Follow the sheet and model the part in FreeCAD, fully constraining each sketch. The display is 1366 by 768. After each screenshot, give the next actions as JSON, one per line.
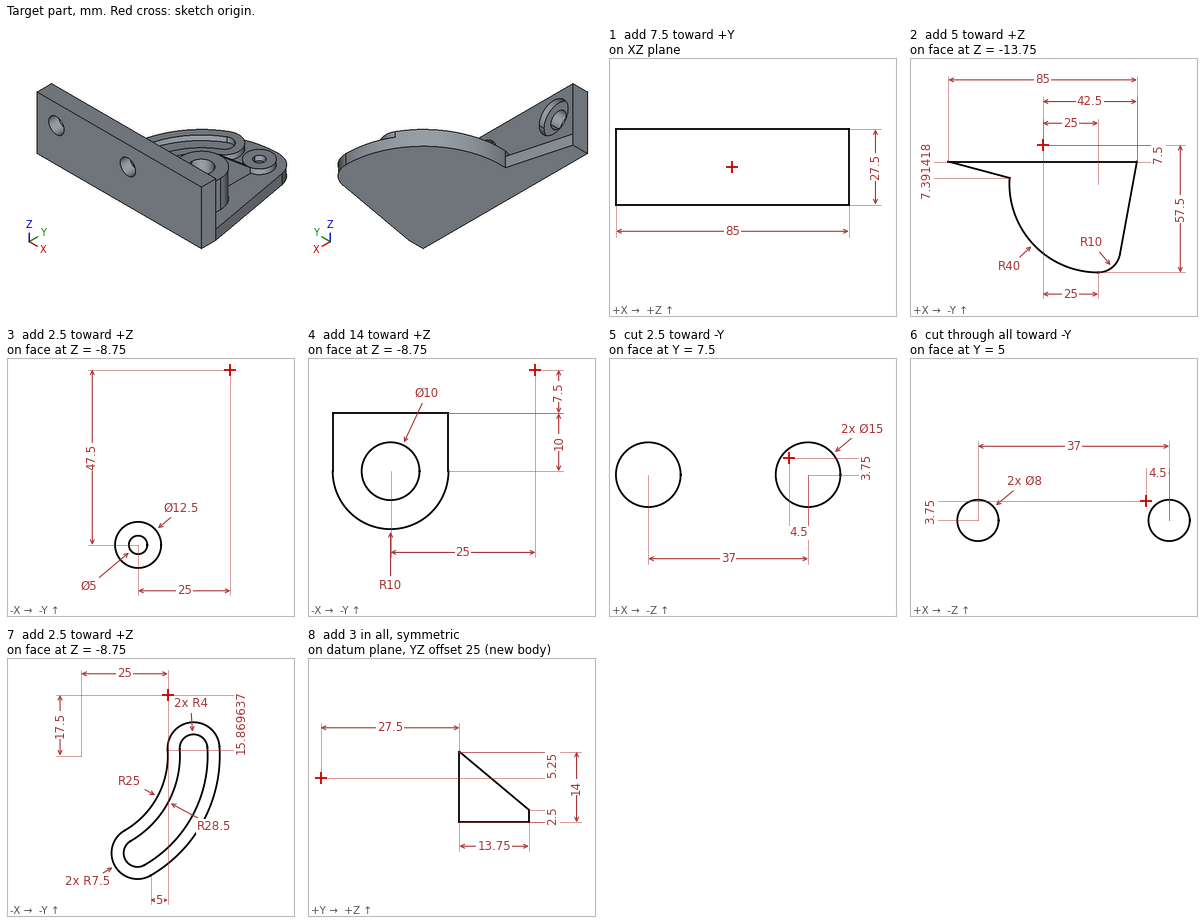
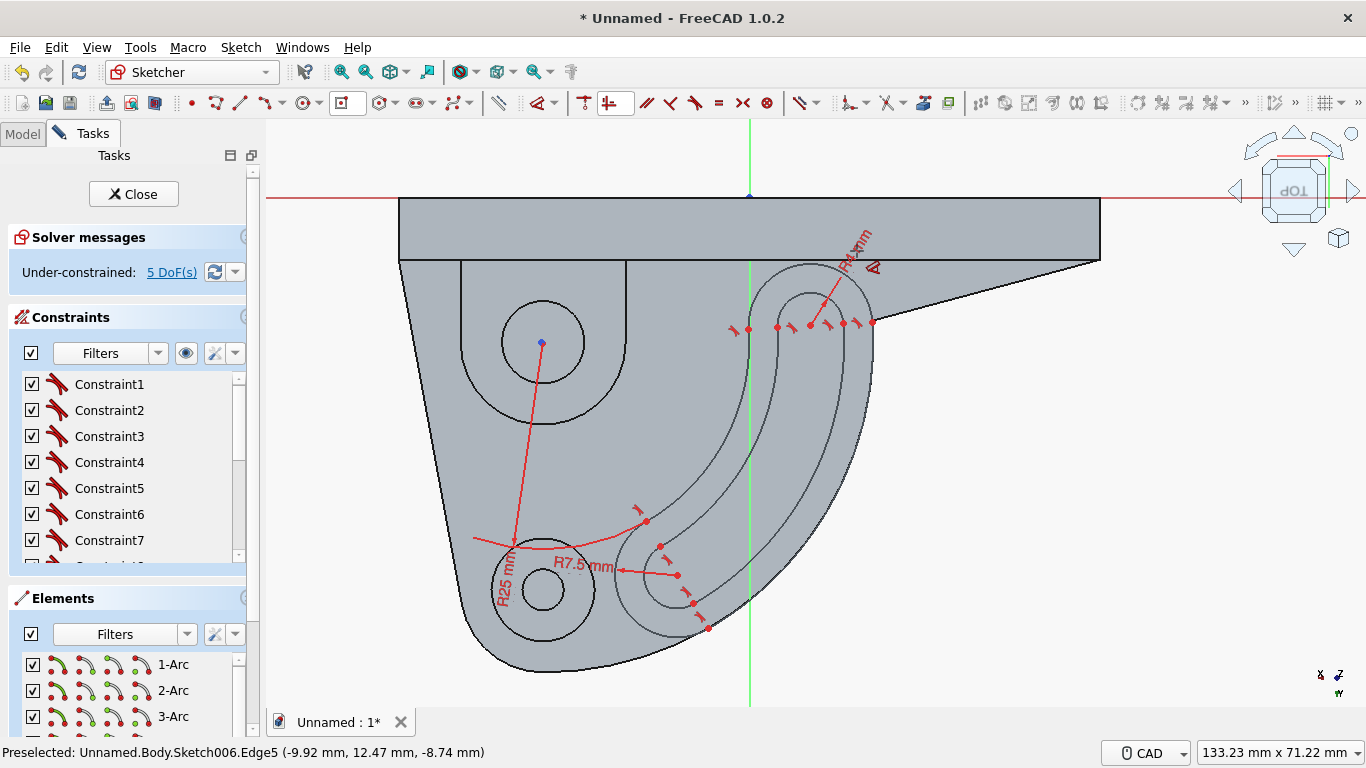
{"action": "left_click", "coordinate": [720, 497]}
{"action": "left_click", "coordinate": [804, 399]}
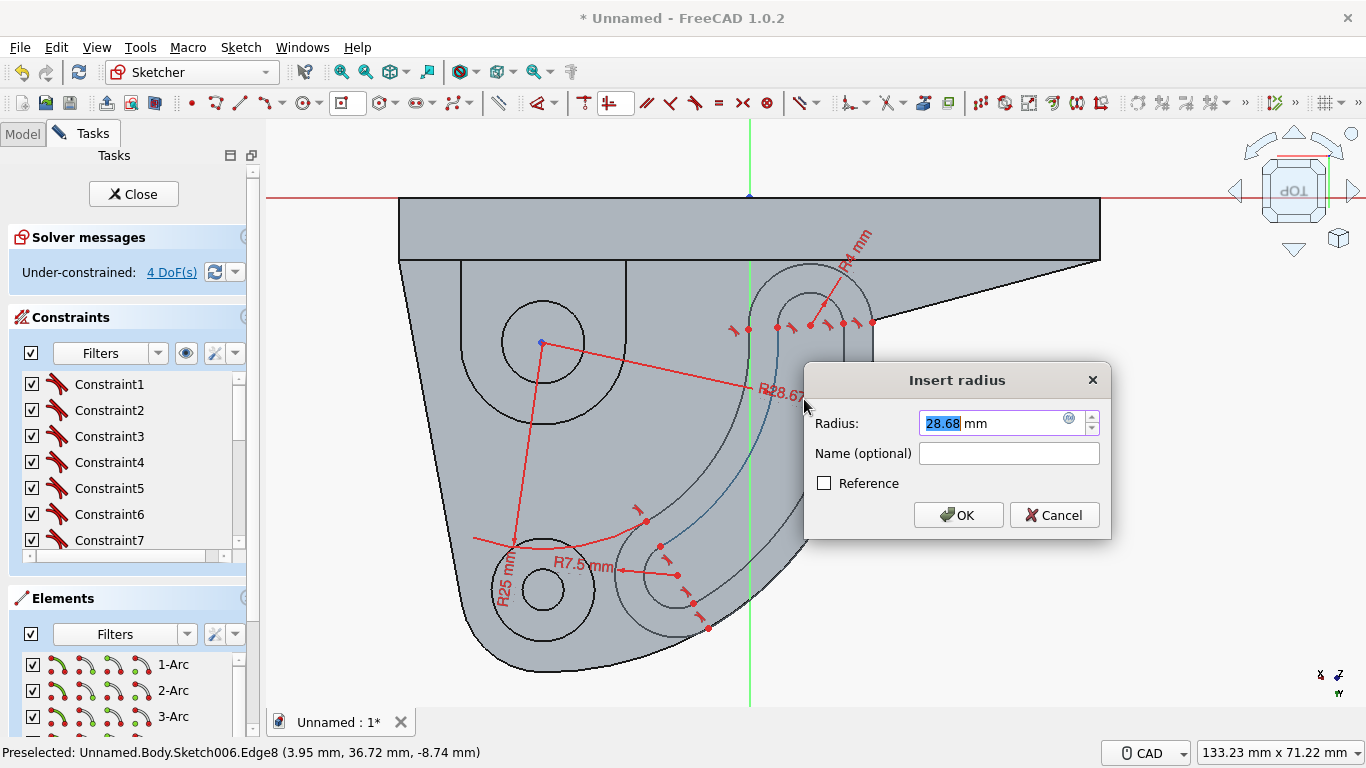
{"action": "type", "text": "28.5"}
{"action": "key", "text": "Return"}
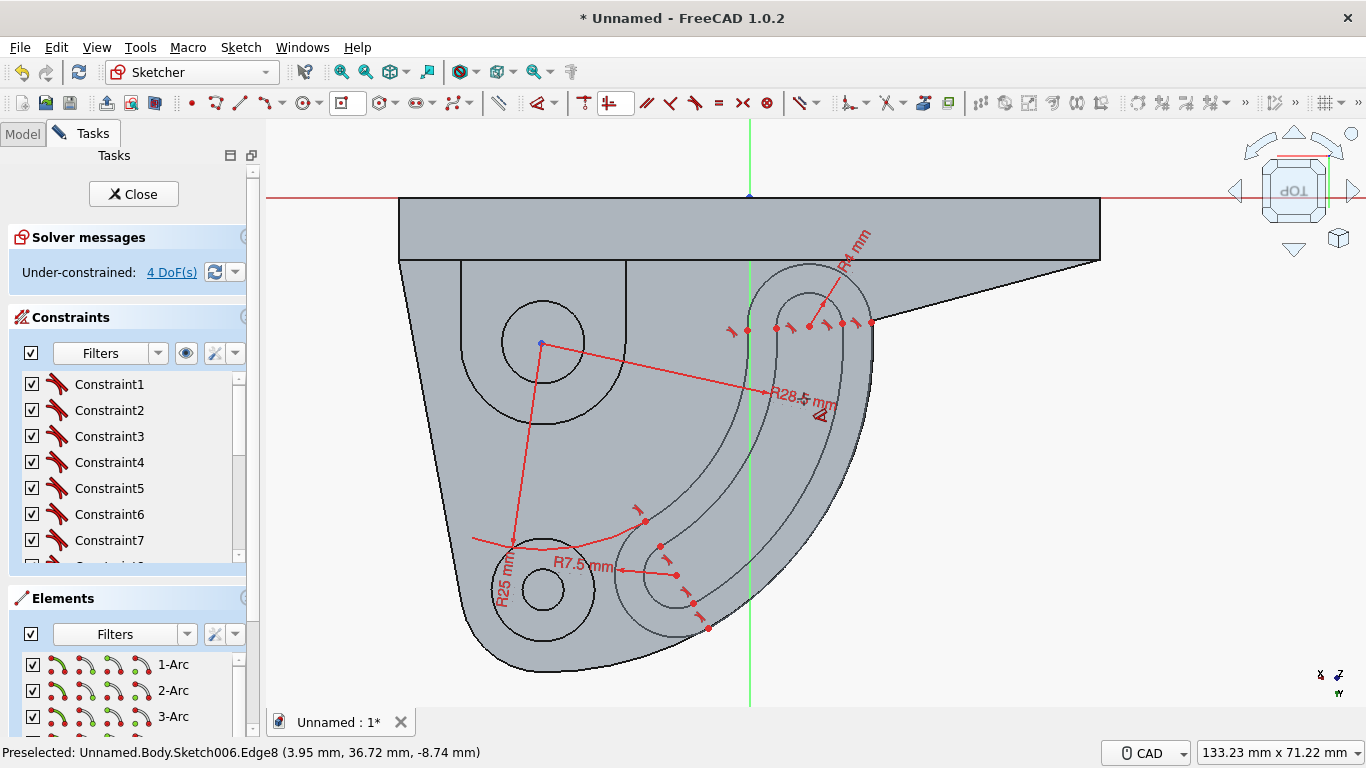
{"action": "left_click", "coordinate": [708, 629]}
{"action": "left_click", "coordinate": [729, 663]}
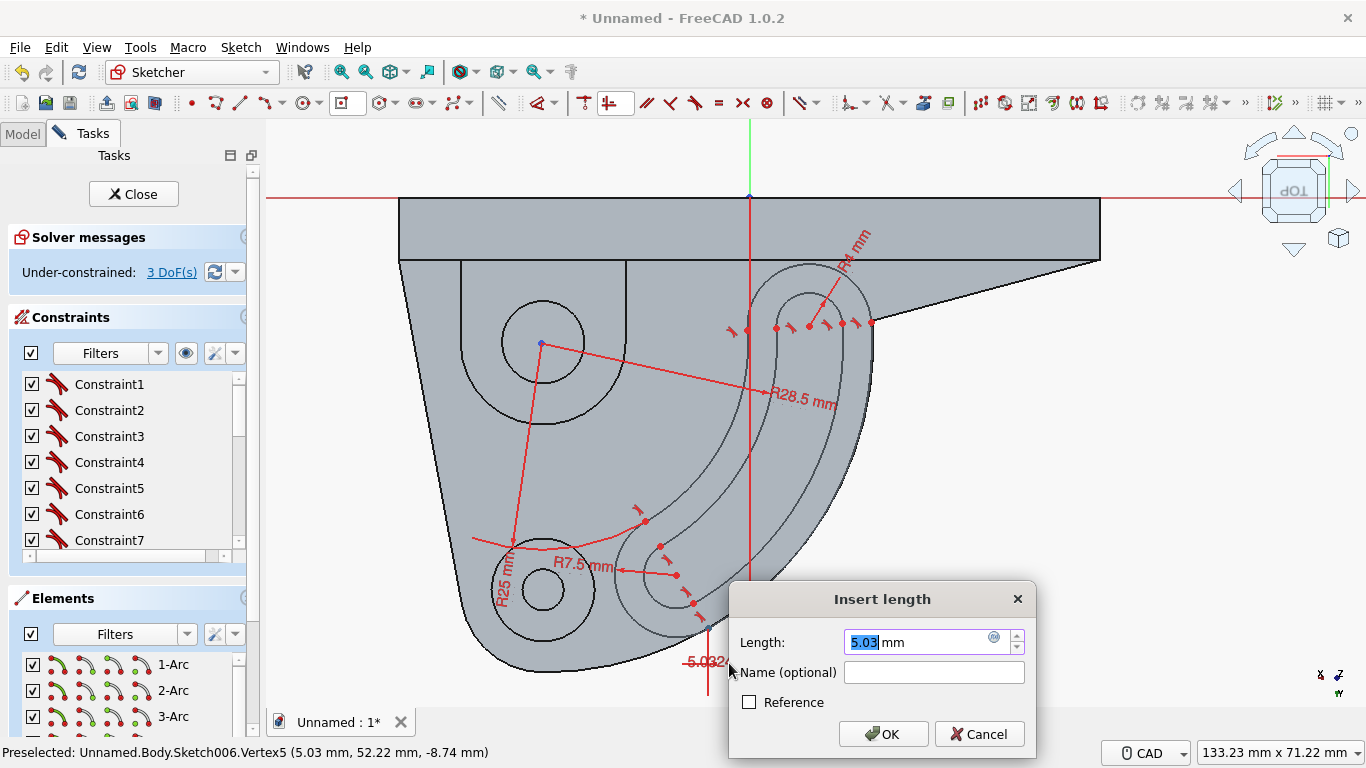
{"action": "type", "text": "5"}
{"action": "key", "text": "Return"}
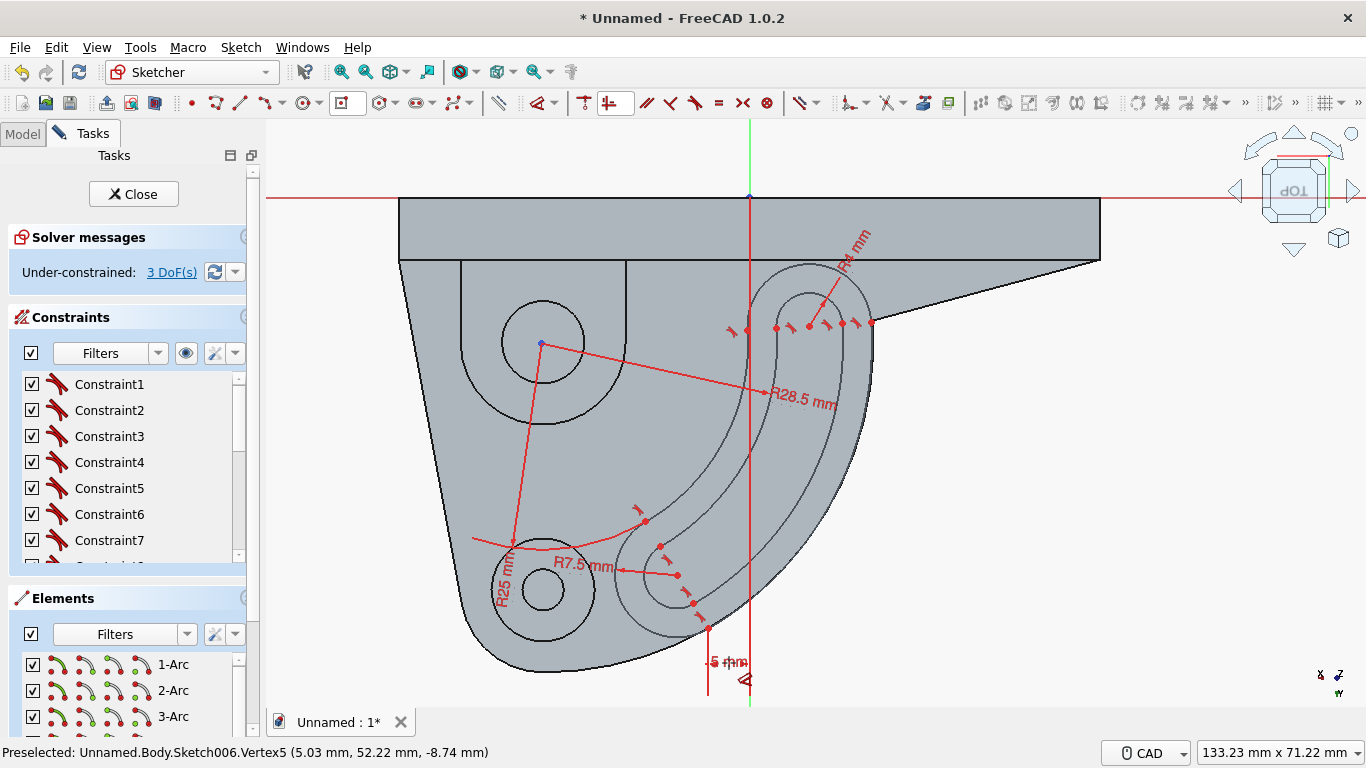
{"action": "left_click", "coordinate": [542, 344]}
{"action": "left_click", "coordinate": [646, 164]}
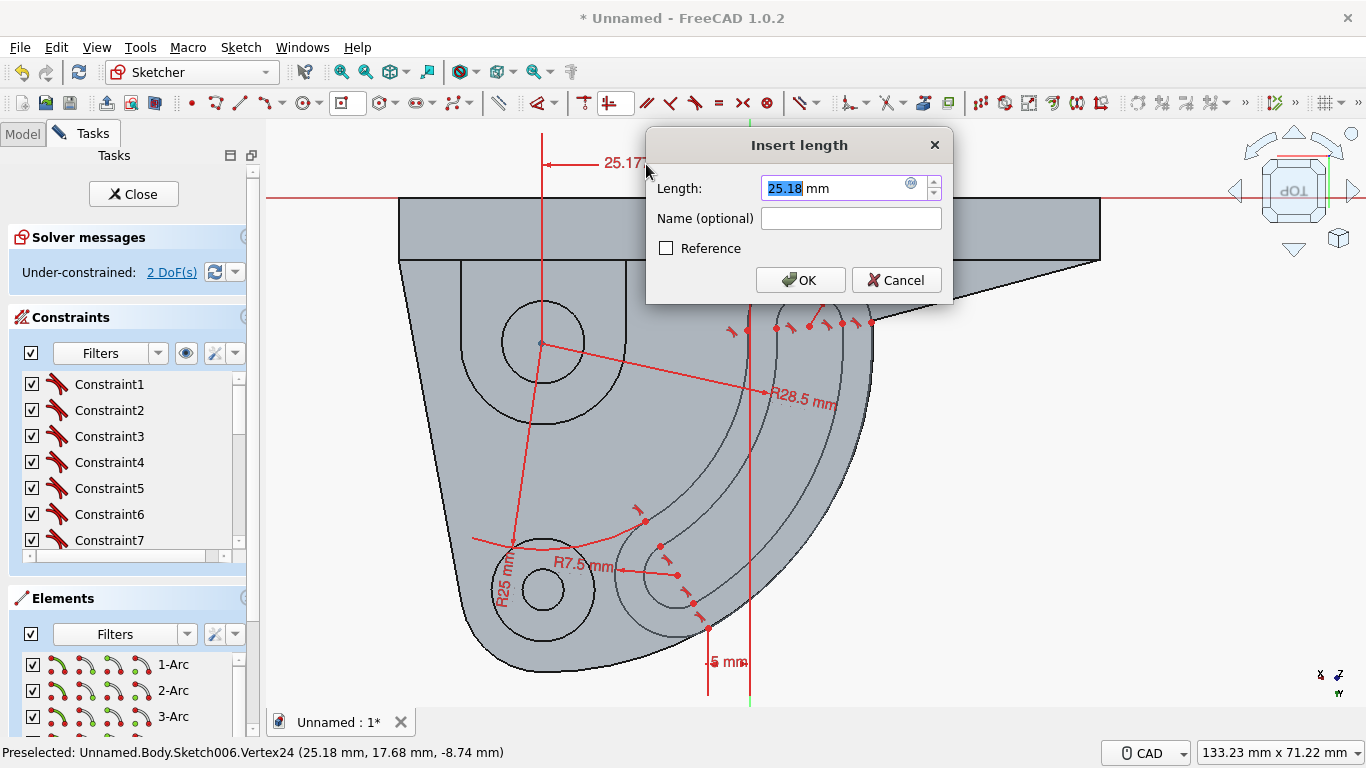
{"action": "type", "text": "25"}
{"action": "key", "text": "Return"}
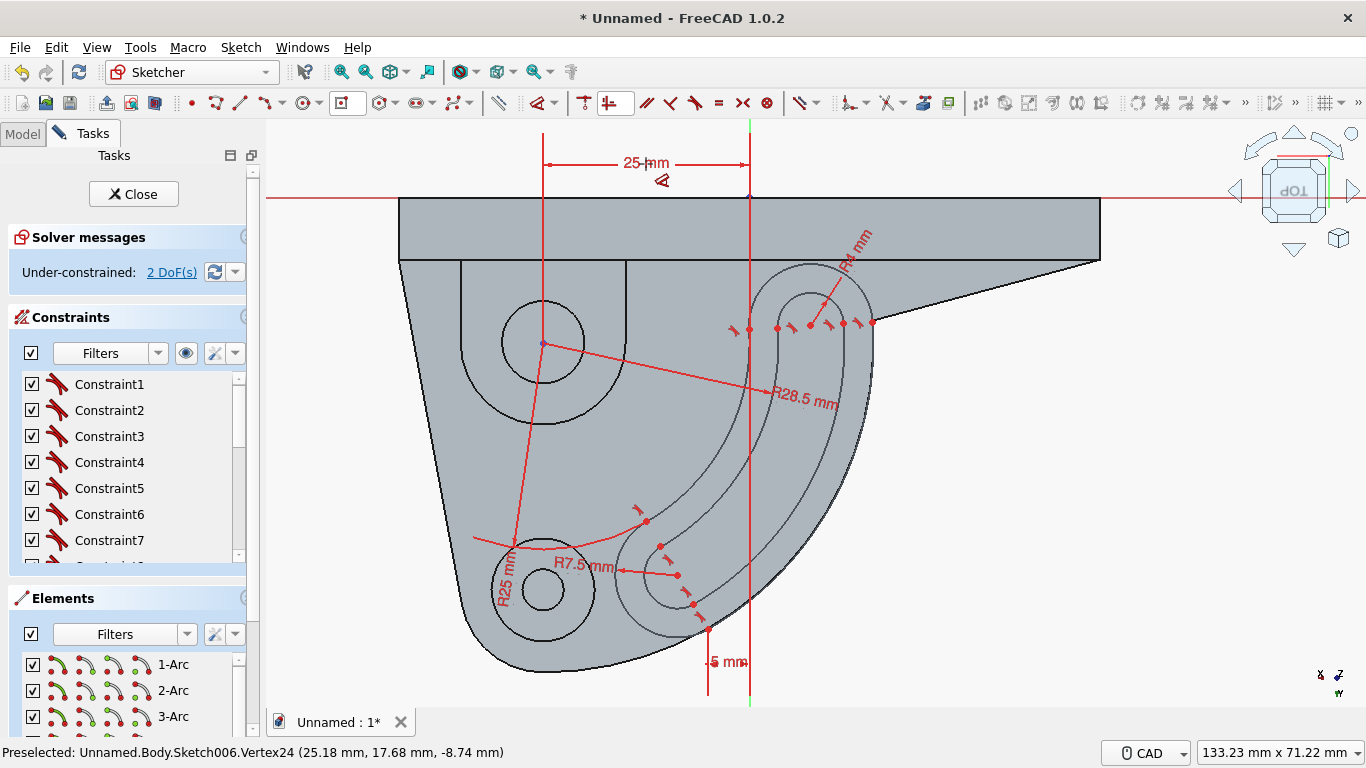
{"action": "left_click", "coordinate": [543, 343]}
{"action": "left_click", "coordinate": [509, 270]}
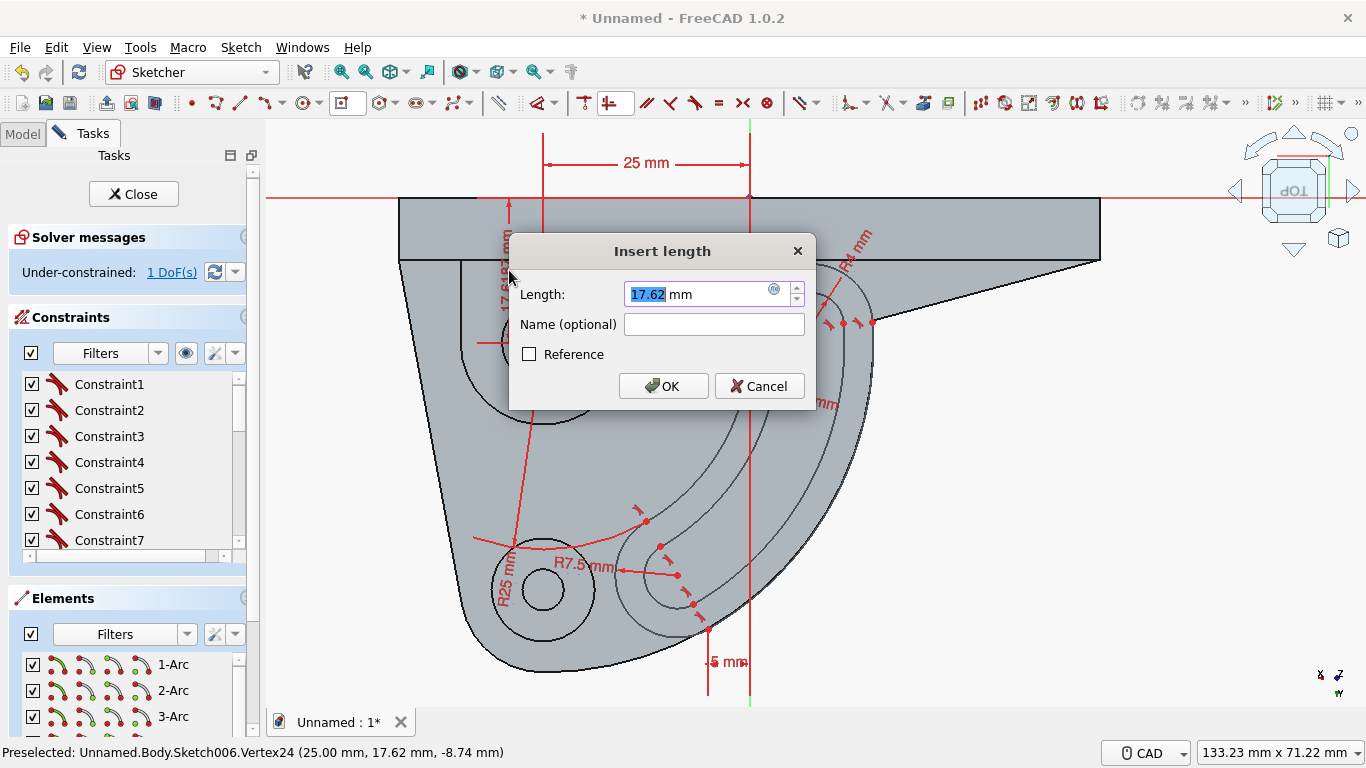
{"action": "type", "text": "17.5"}
{"action": "key", "text": "Return"}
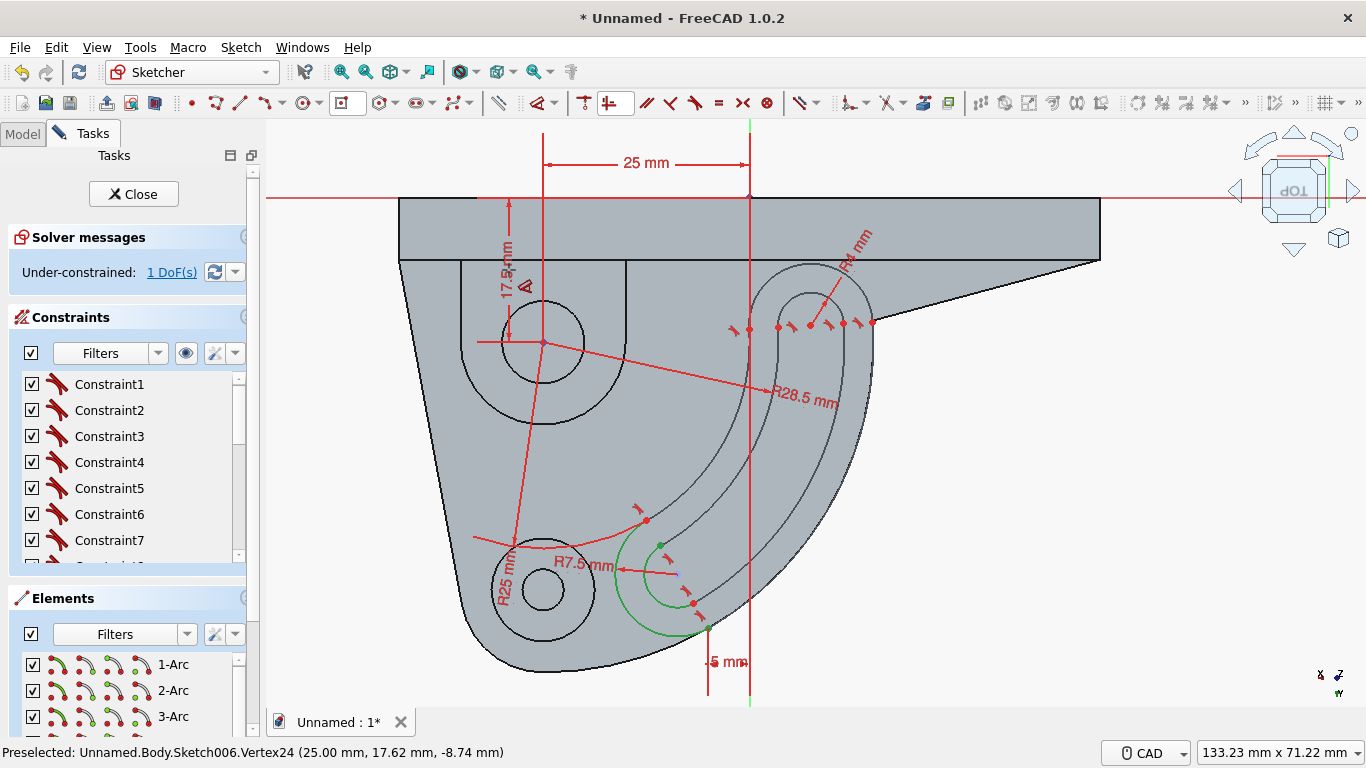
{"action": "left_click", "coordinate": [749, 330]}
{"action": "left_click", "coordinate": [784, 233]}